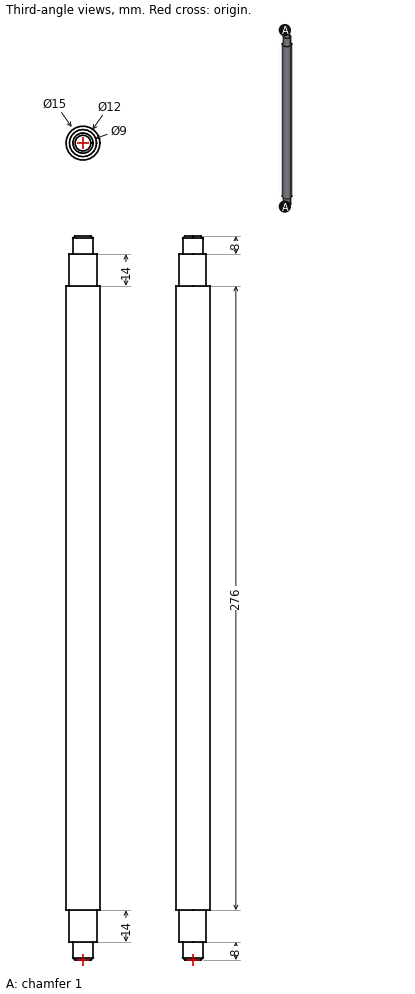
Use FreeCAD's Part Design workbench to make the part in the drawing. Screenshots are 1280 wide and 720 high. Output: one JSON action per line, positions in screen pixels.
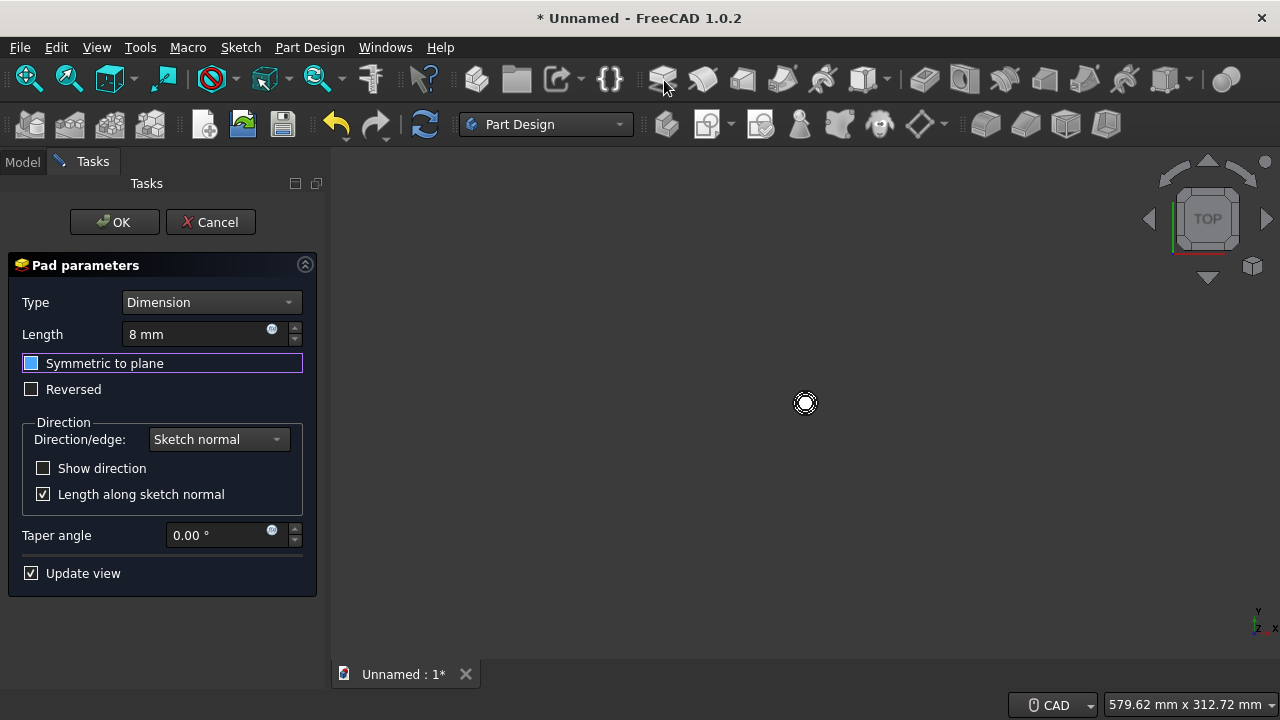
{"action": "left_click", "coordinate": [115, 222]}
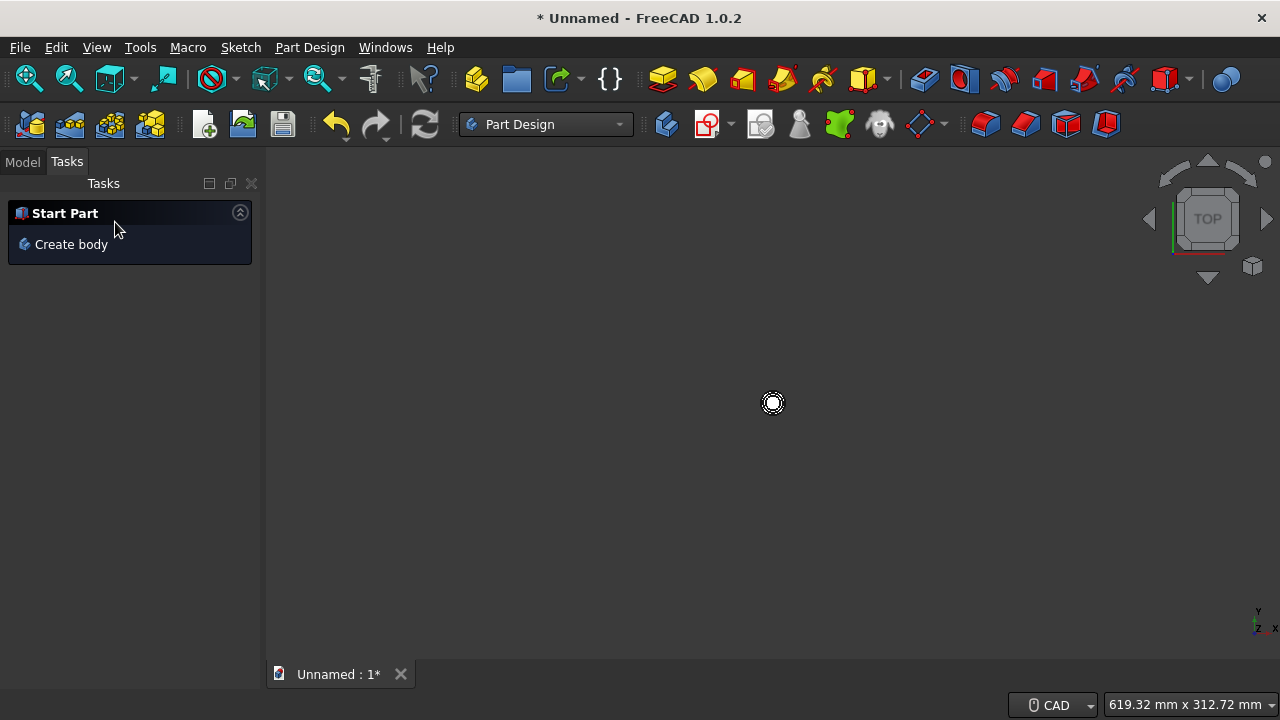
{"action": "key", "text": "v f"}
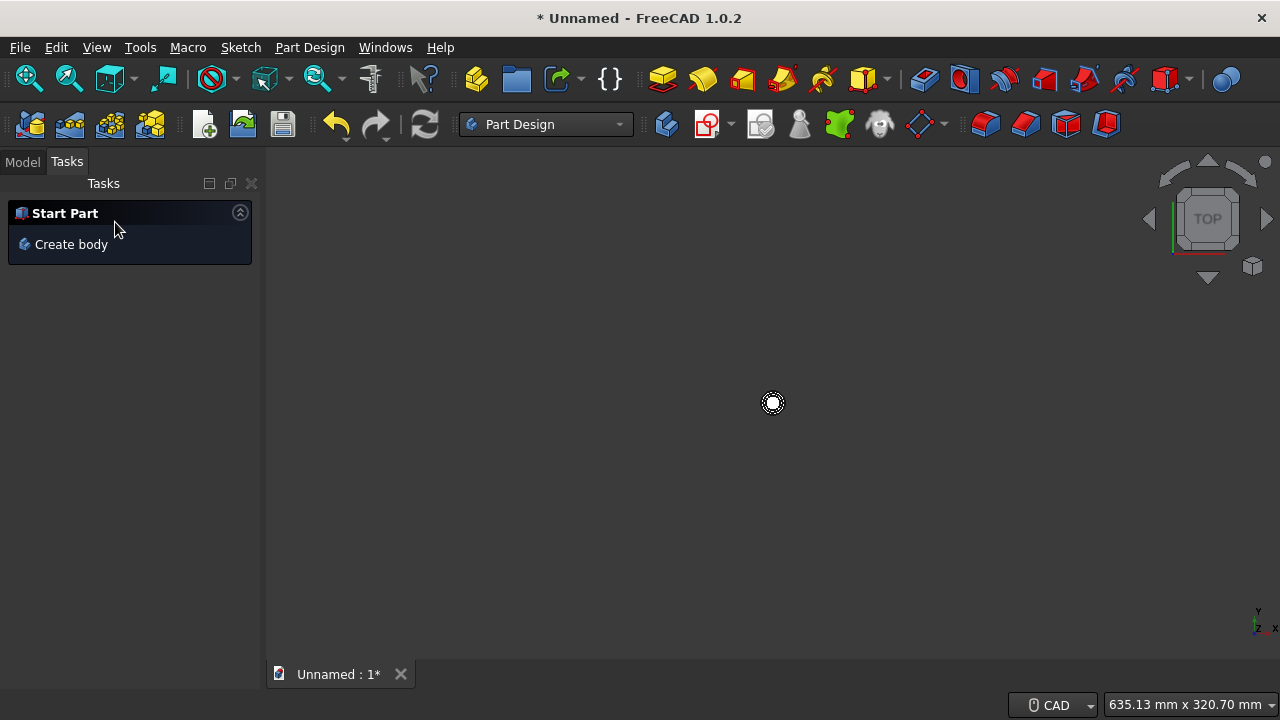
{"action": "left_click", "coordinate": [766, 402]}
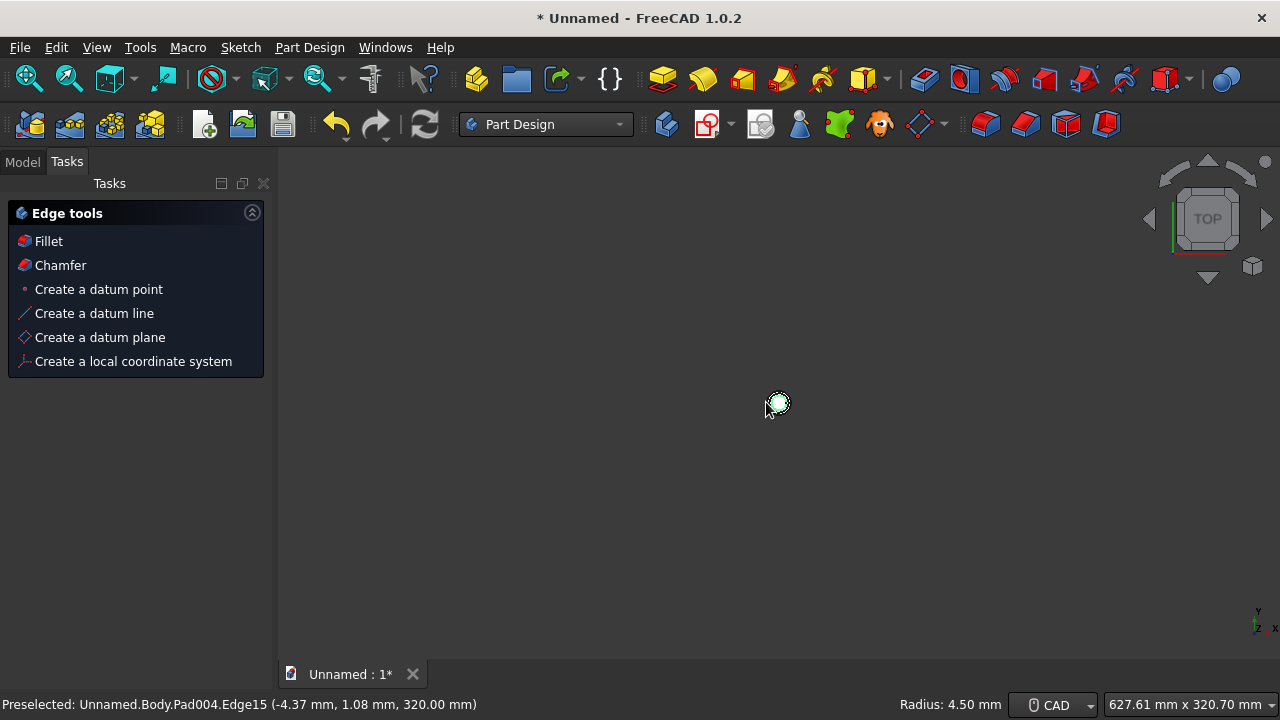
{"action": "key", "text": "0"}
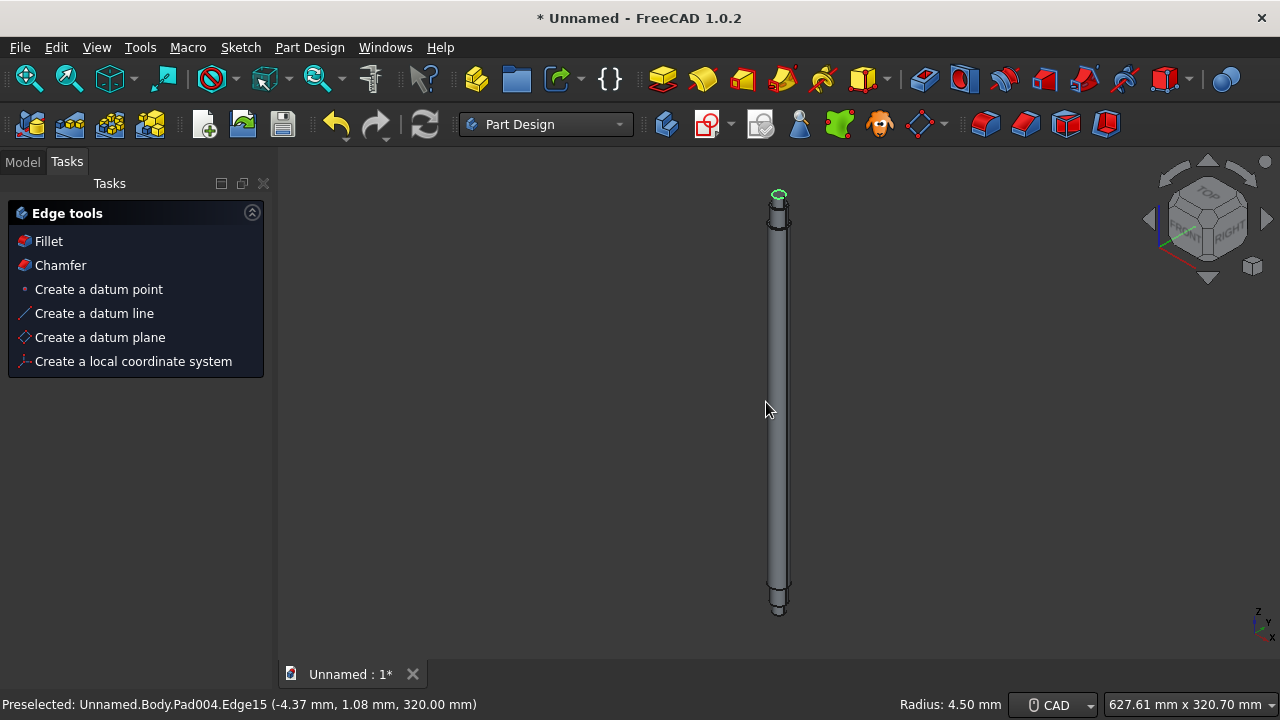
{"action": "key", "text": "2"}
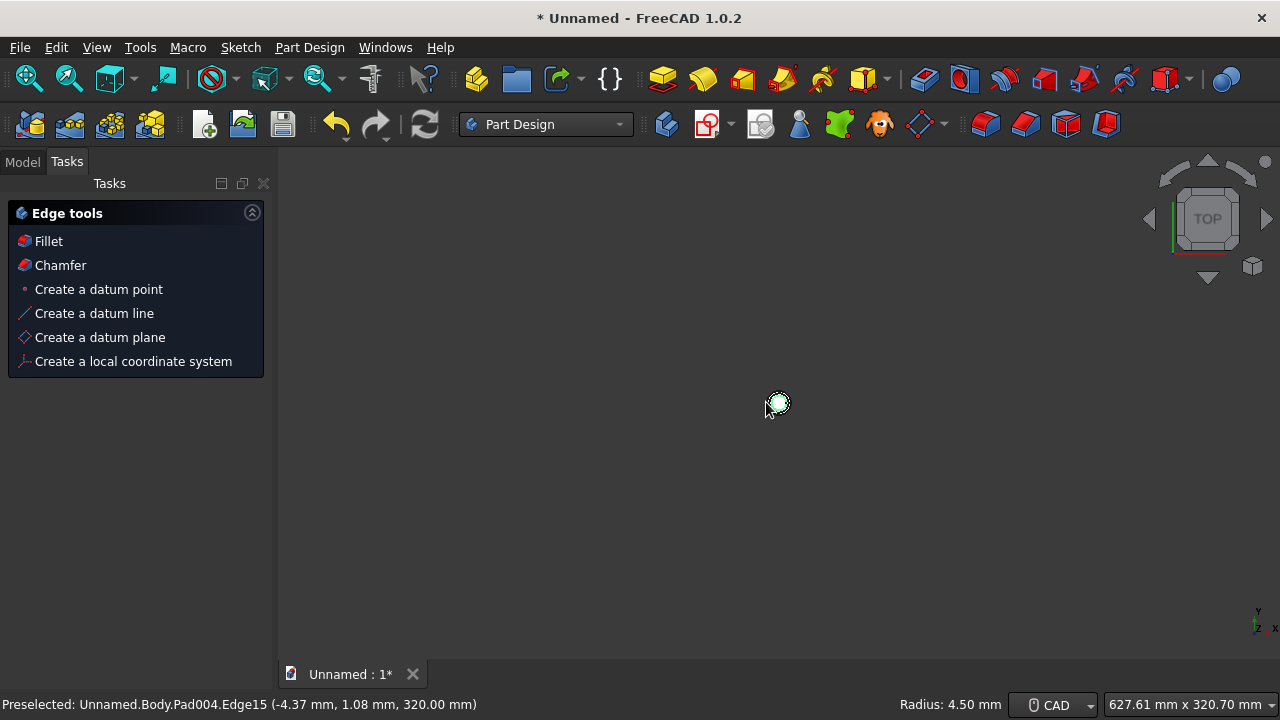
{"action": "key", "text": "v f"}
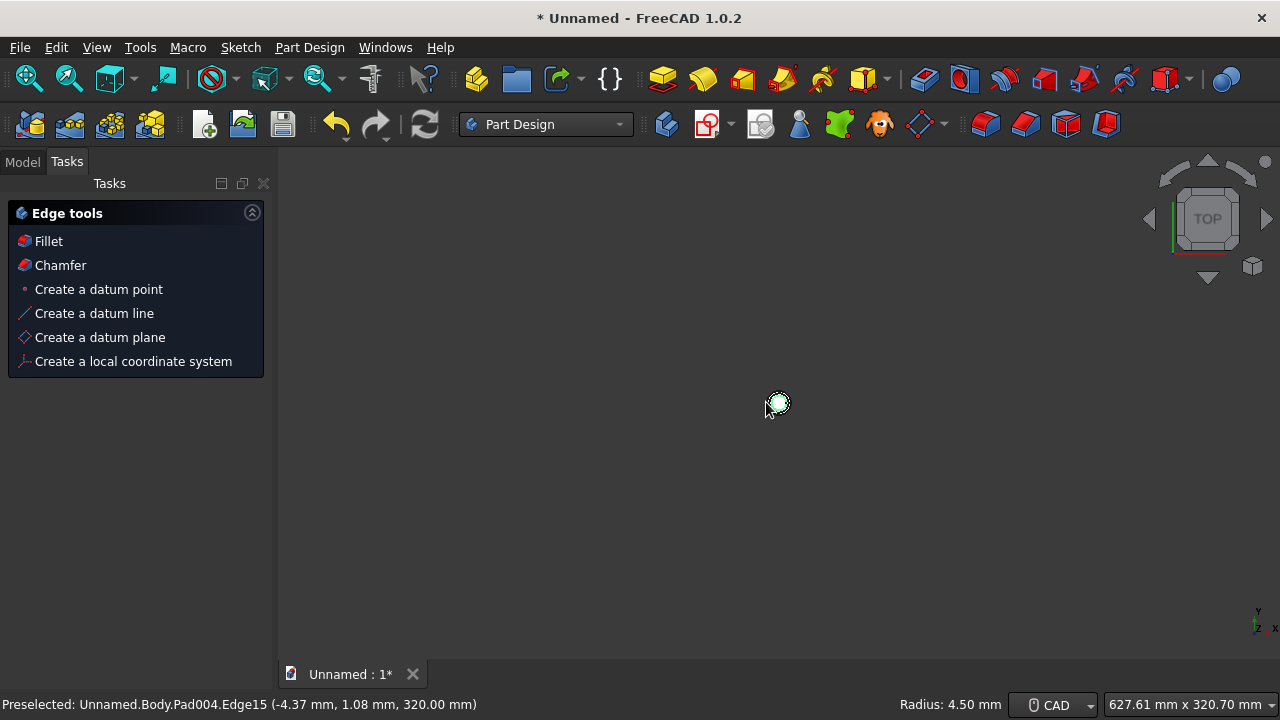
{"action": "key", "text": "1"}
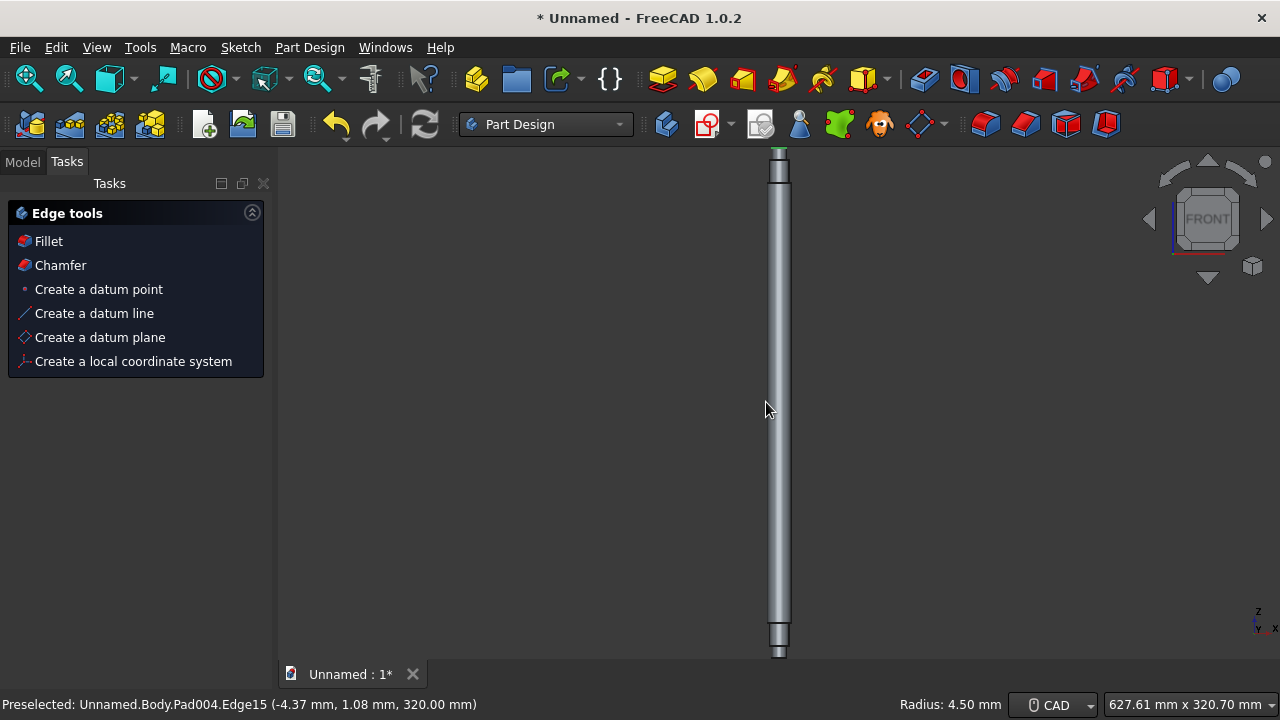
{"action": "key", "text": "3"}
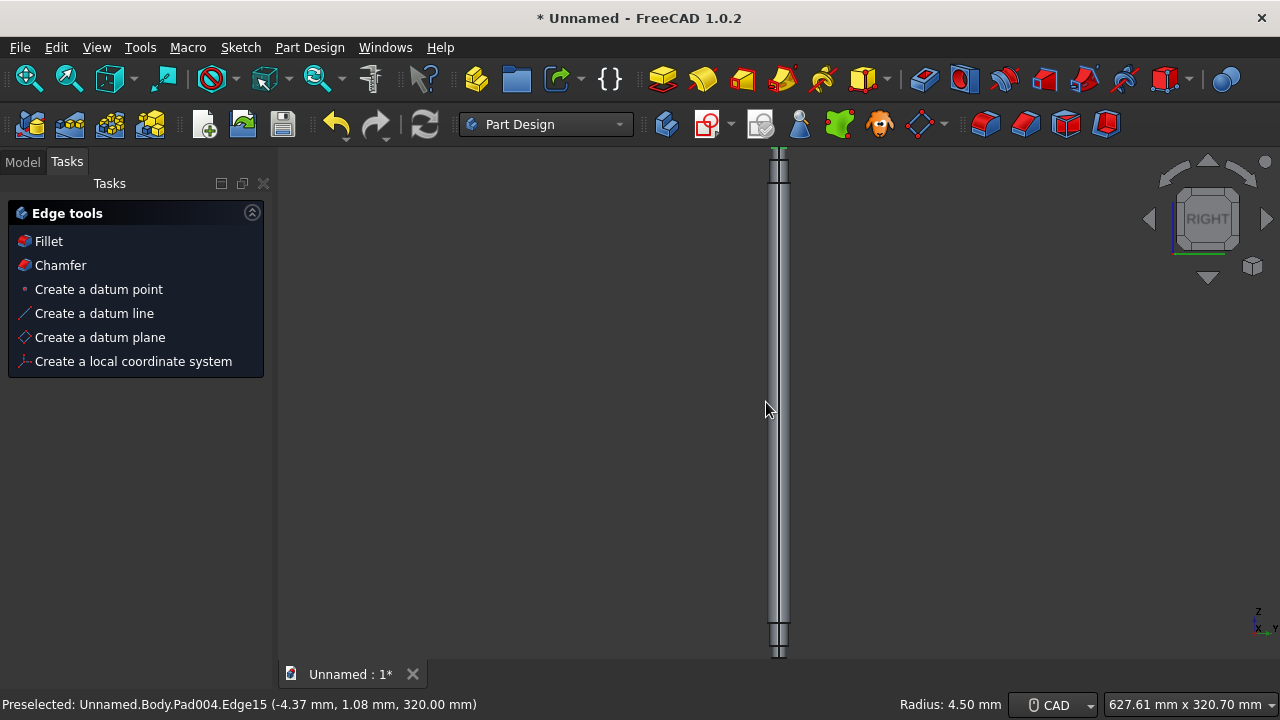
{"action": "key", "text": "5"}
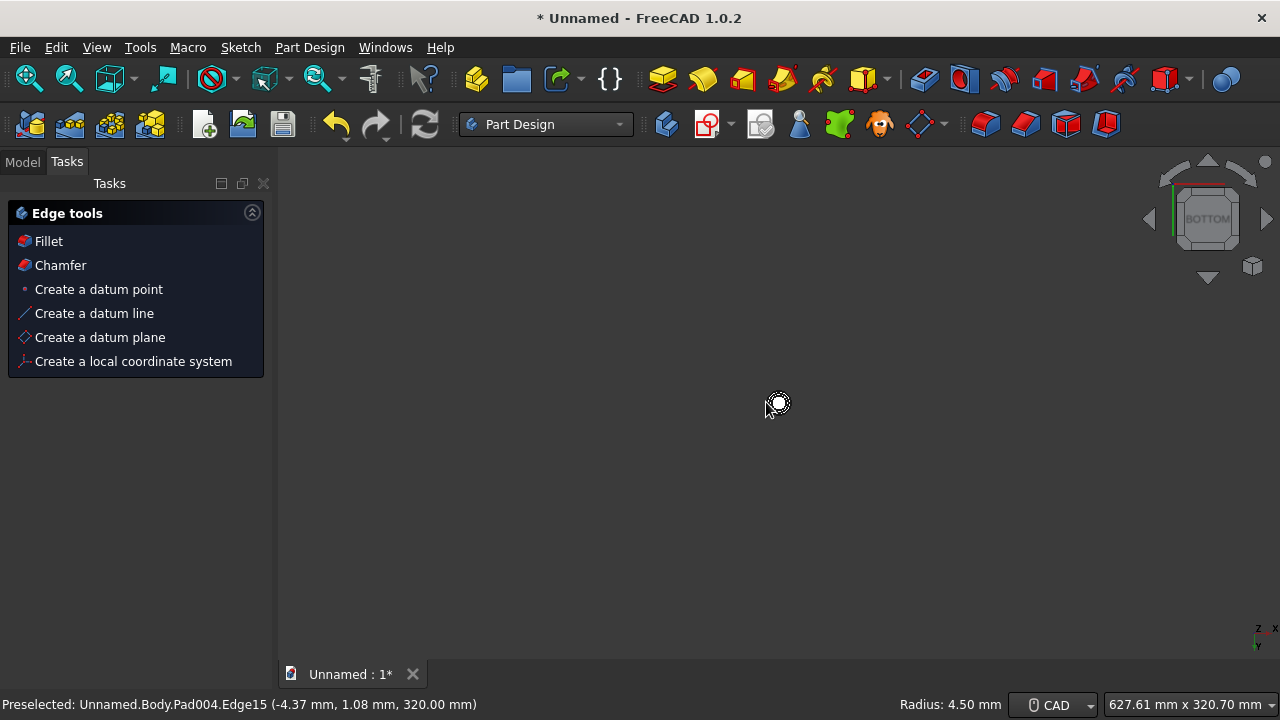
{"action": "key", "text": "v f"}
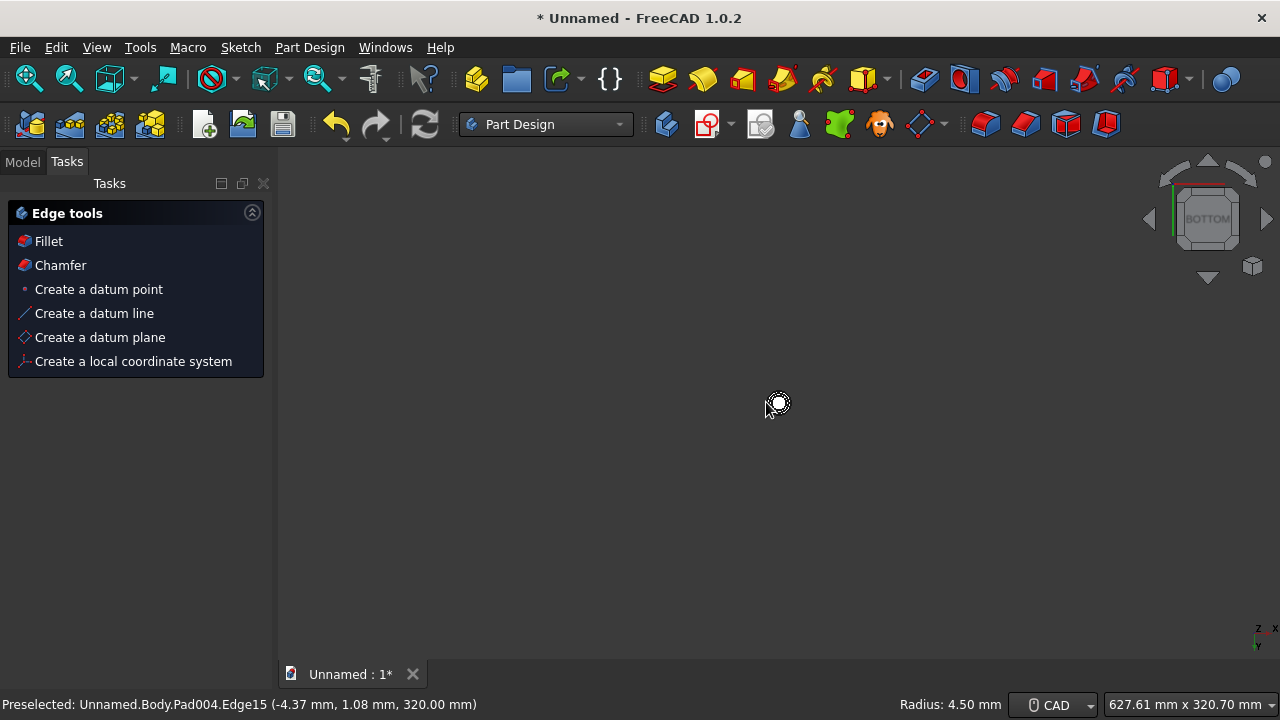
{"action": "left_click", "coordinate": [772, 402], "text": "ctrl"}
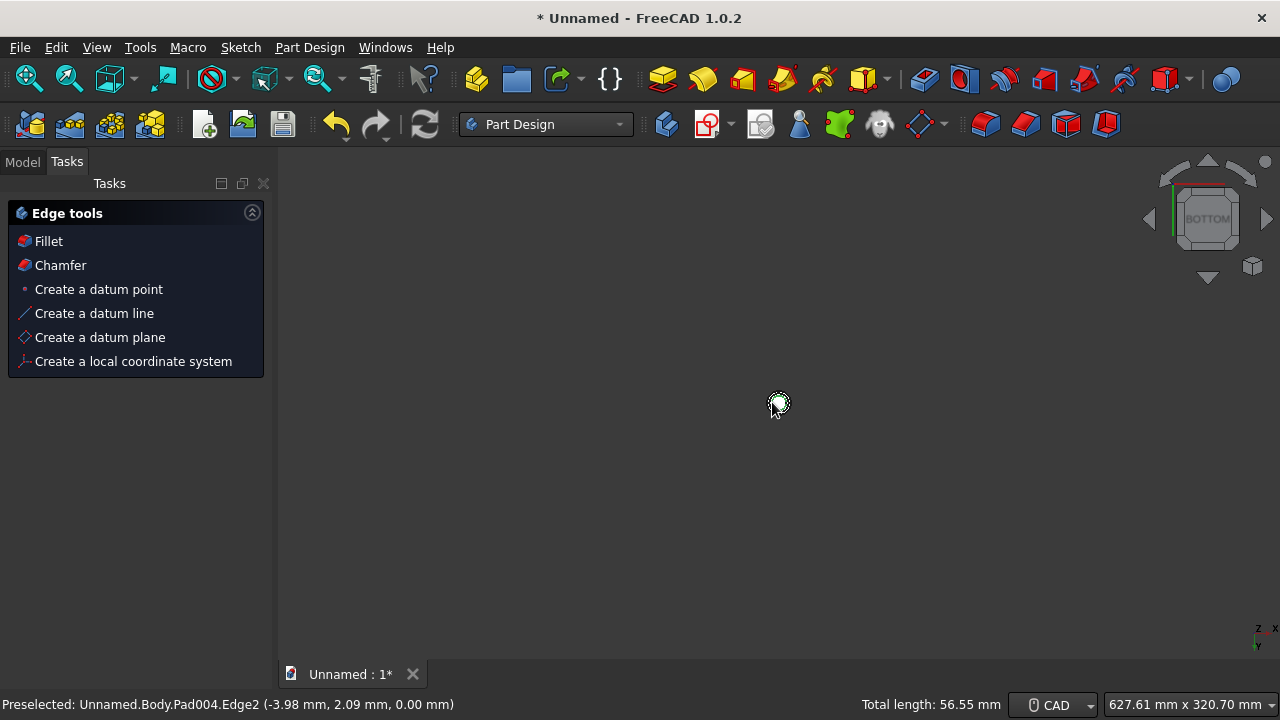
{"action": "left_click", "coordinate": [1026, 124]}